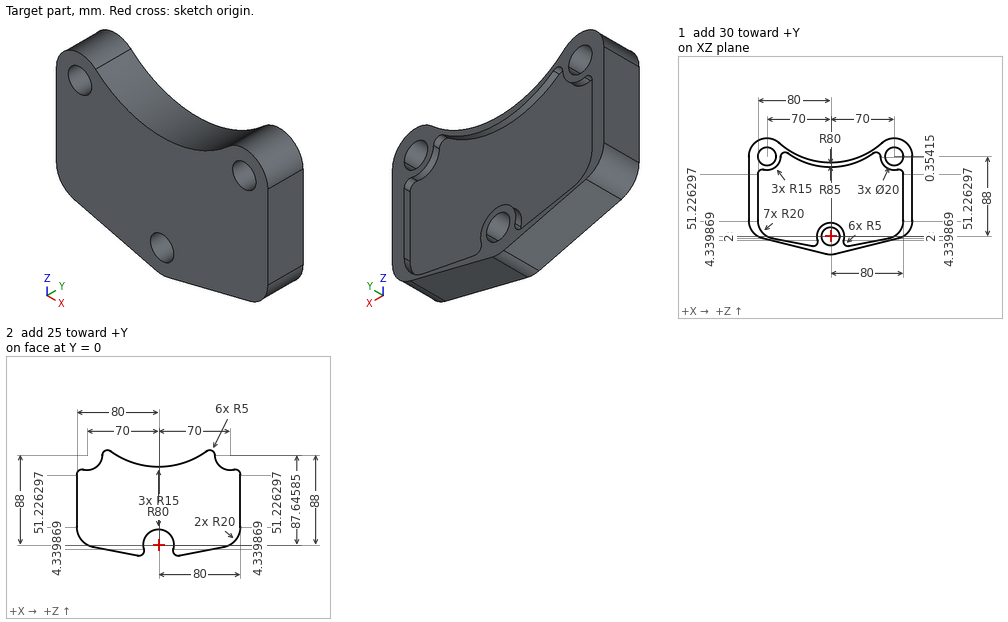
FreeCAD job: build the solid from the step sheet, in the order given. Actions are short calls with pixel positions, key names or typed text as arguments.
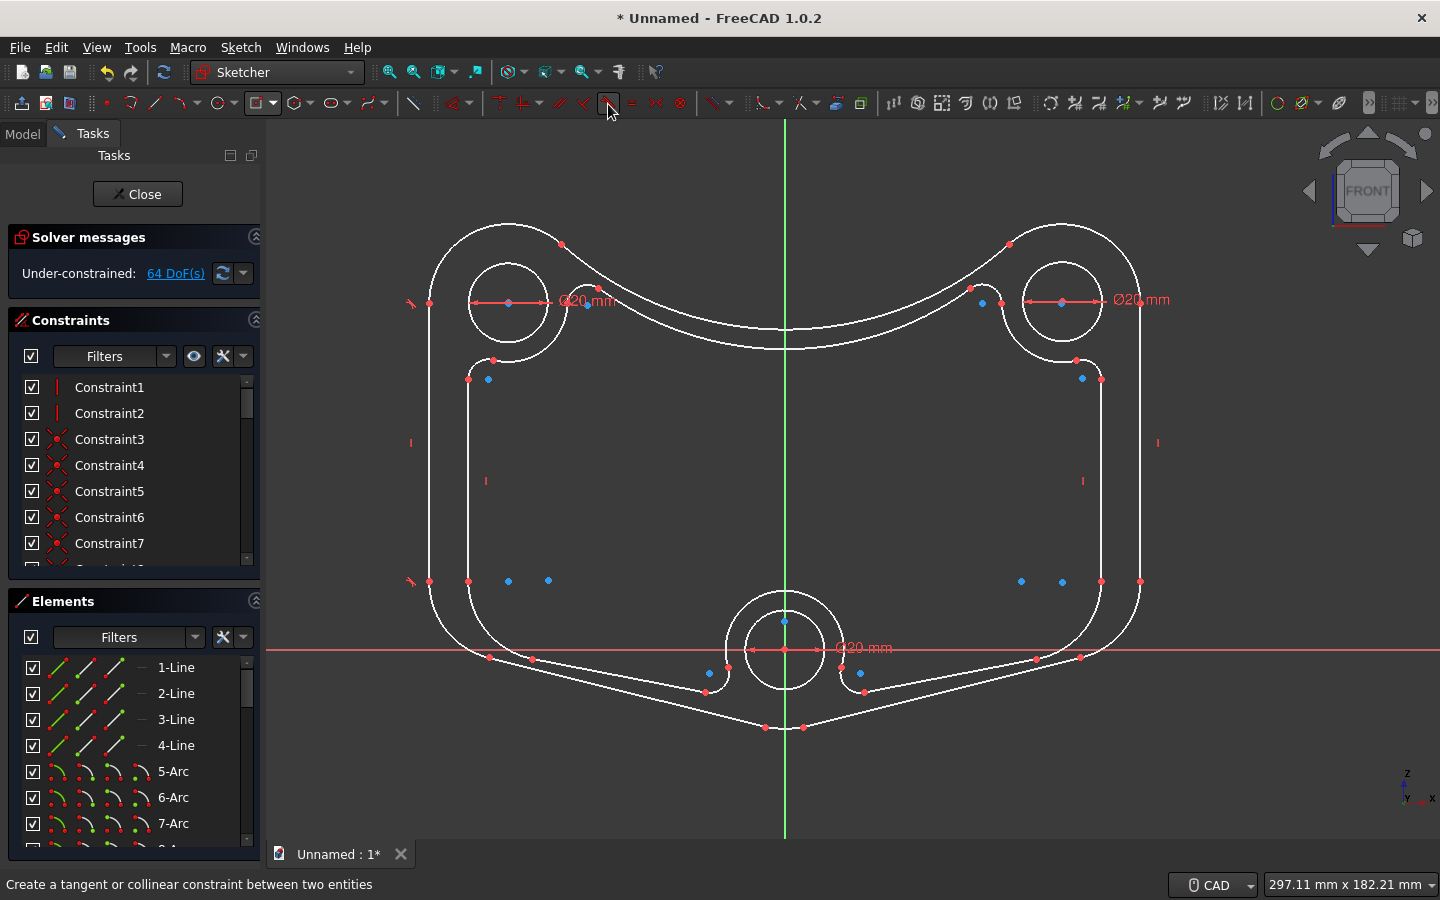
click(1140, 387)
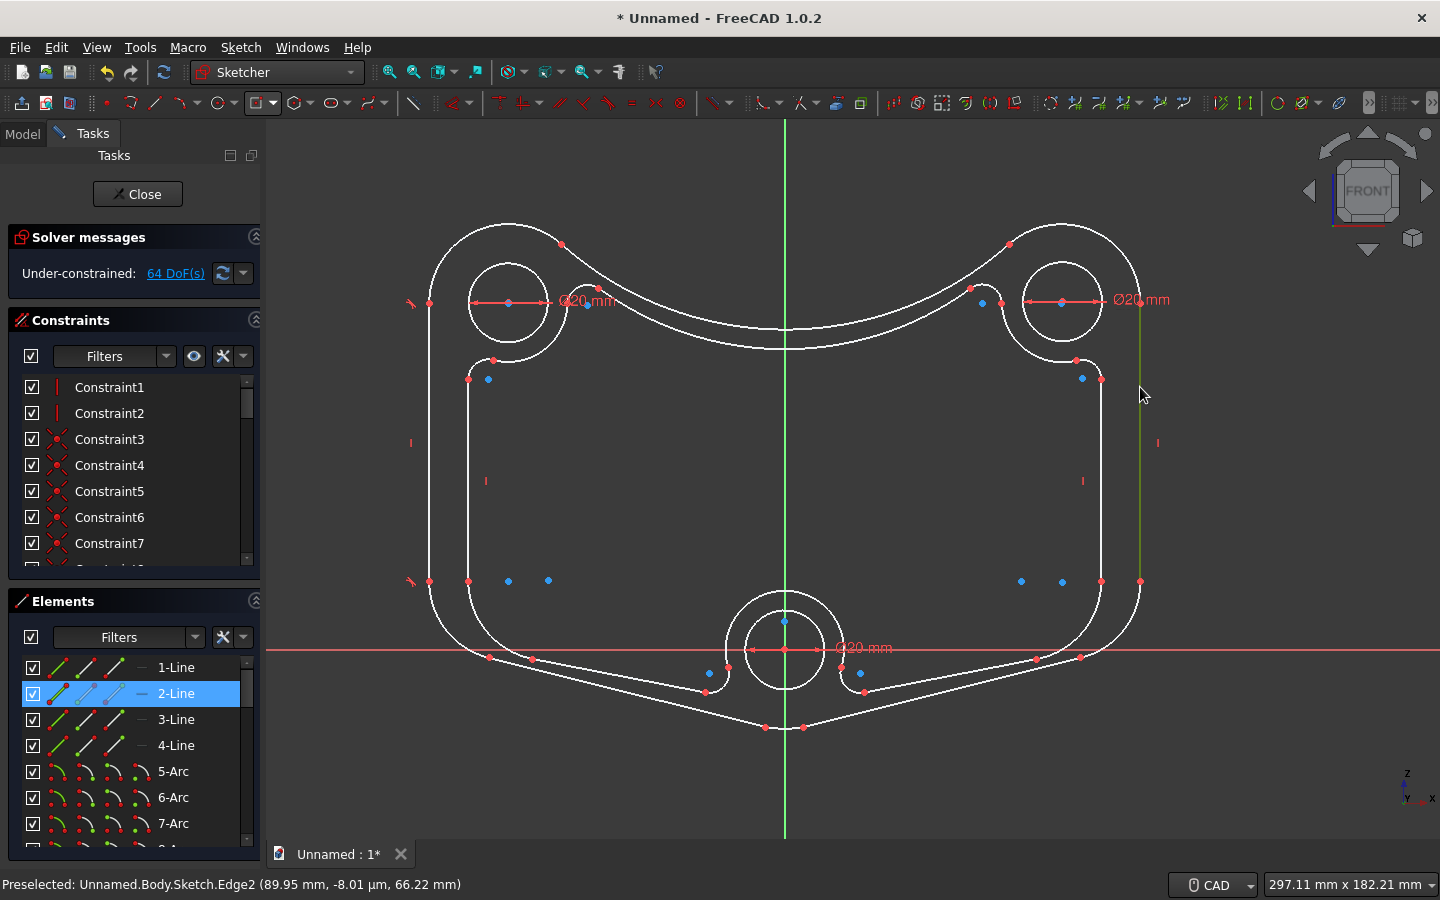
click(1122, 253)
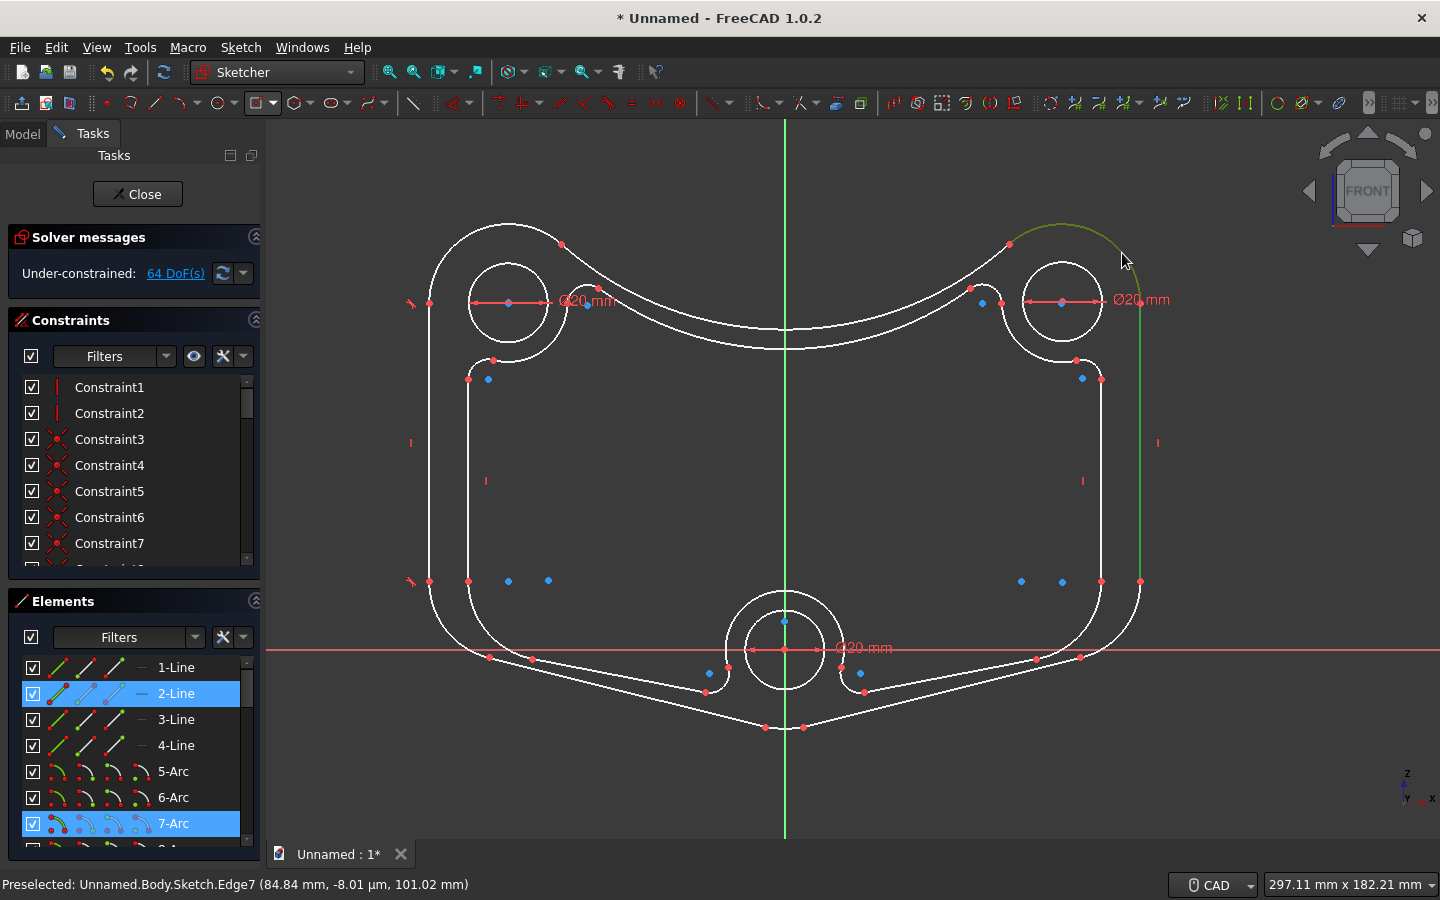
click(608, 104)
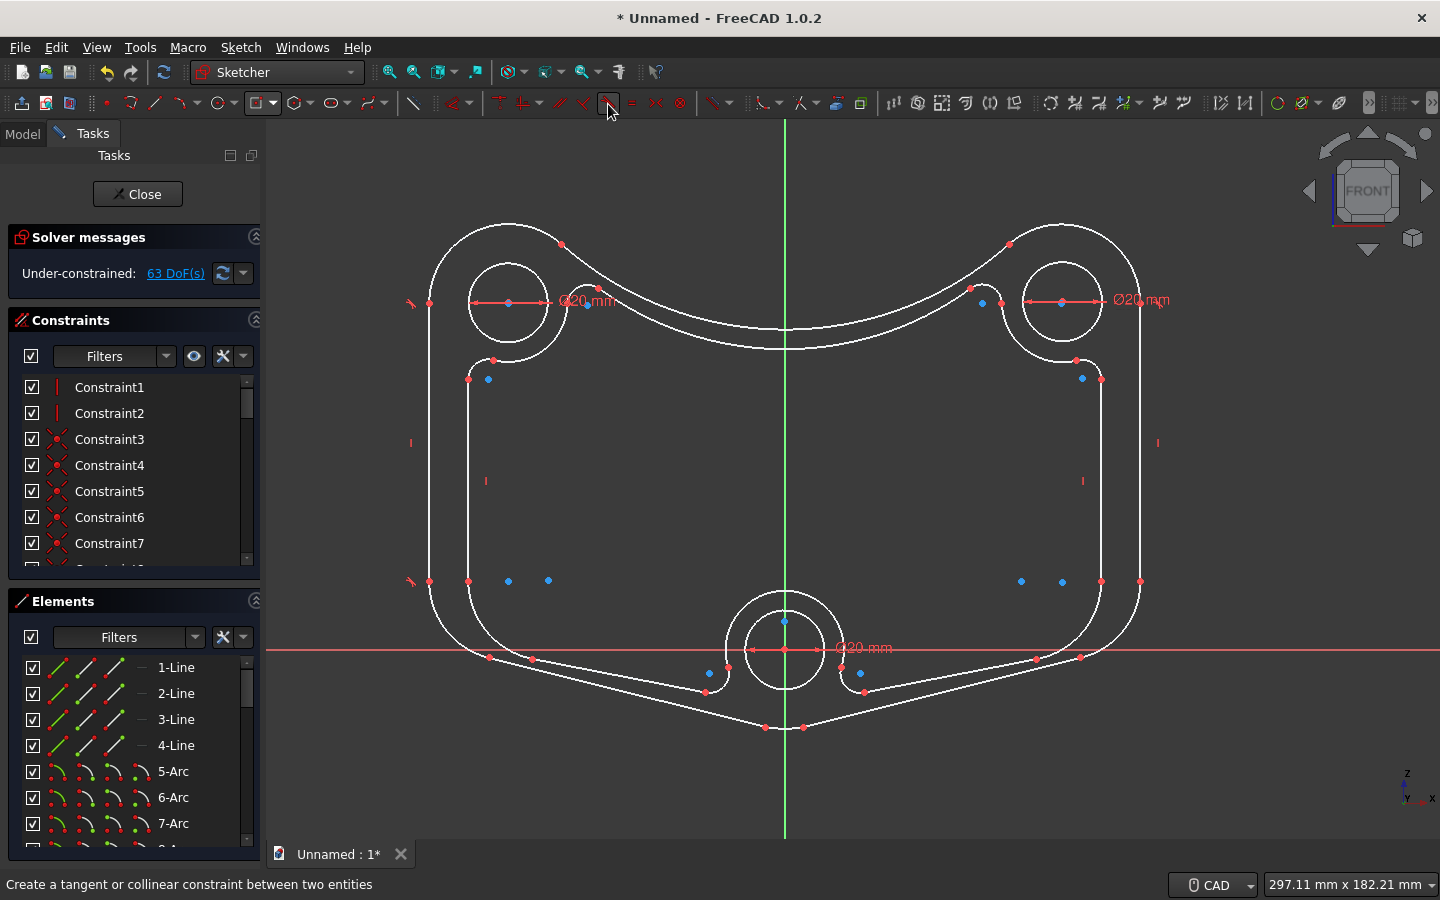
click(1140, 387)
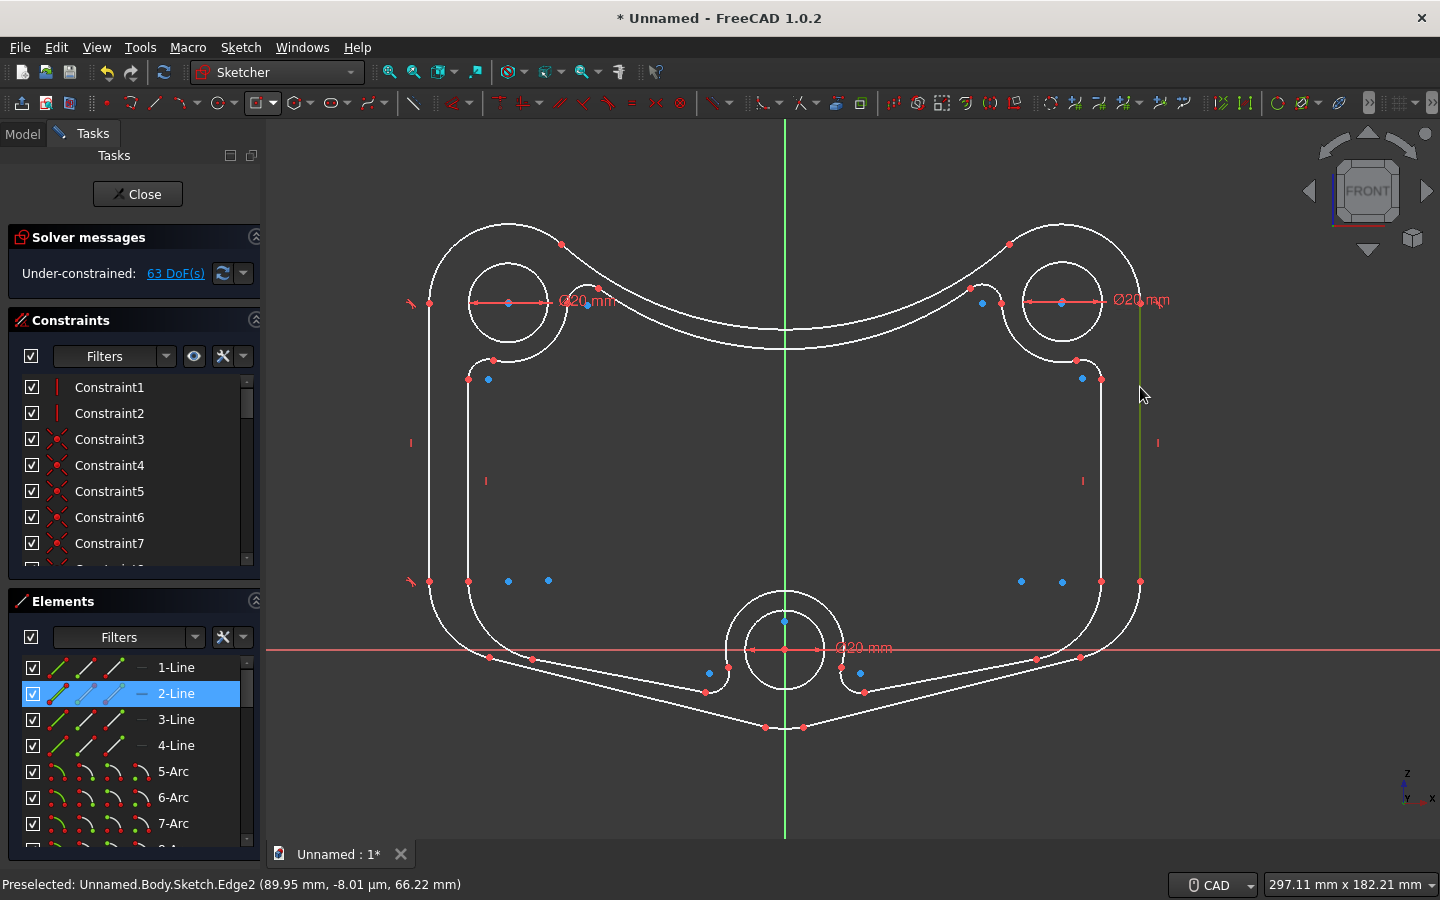
click(1134, 612)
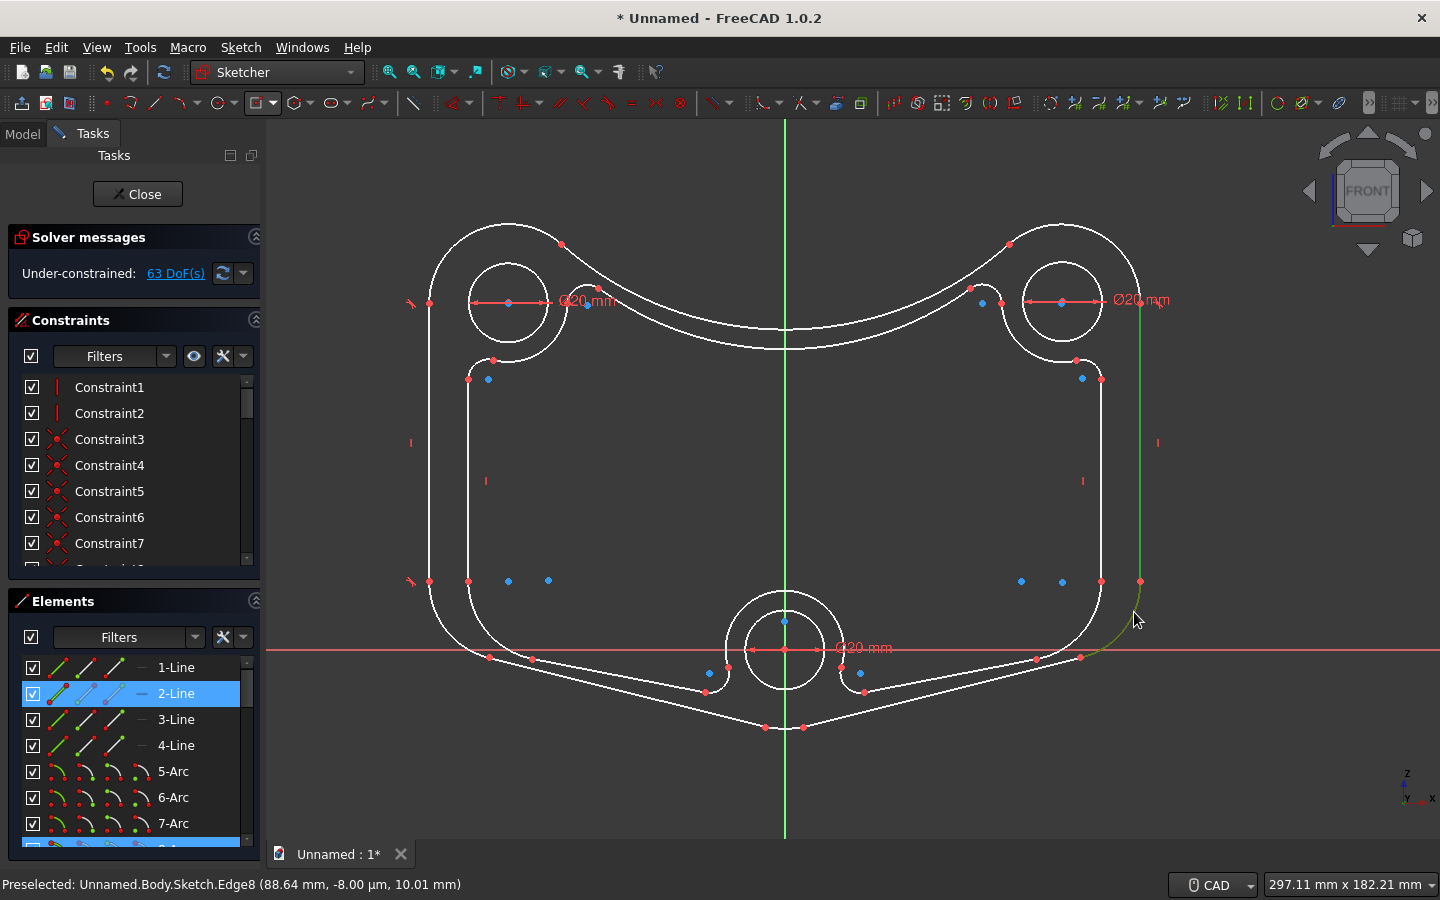
click(608, 104)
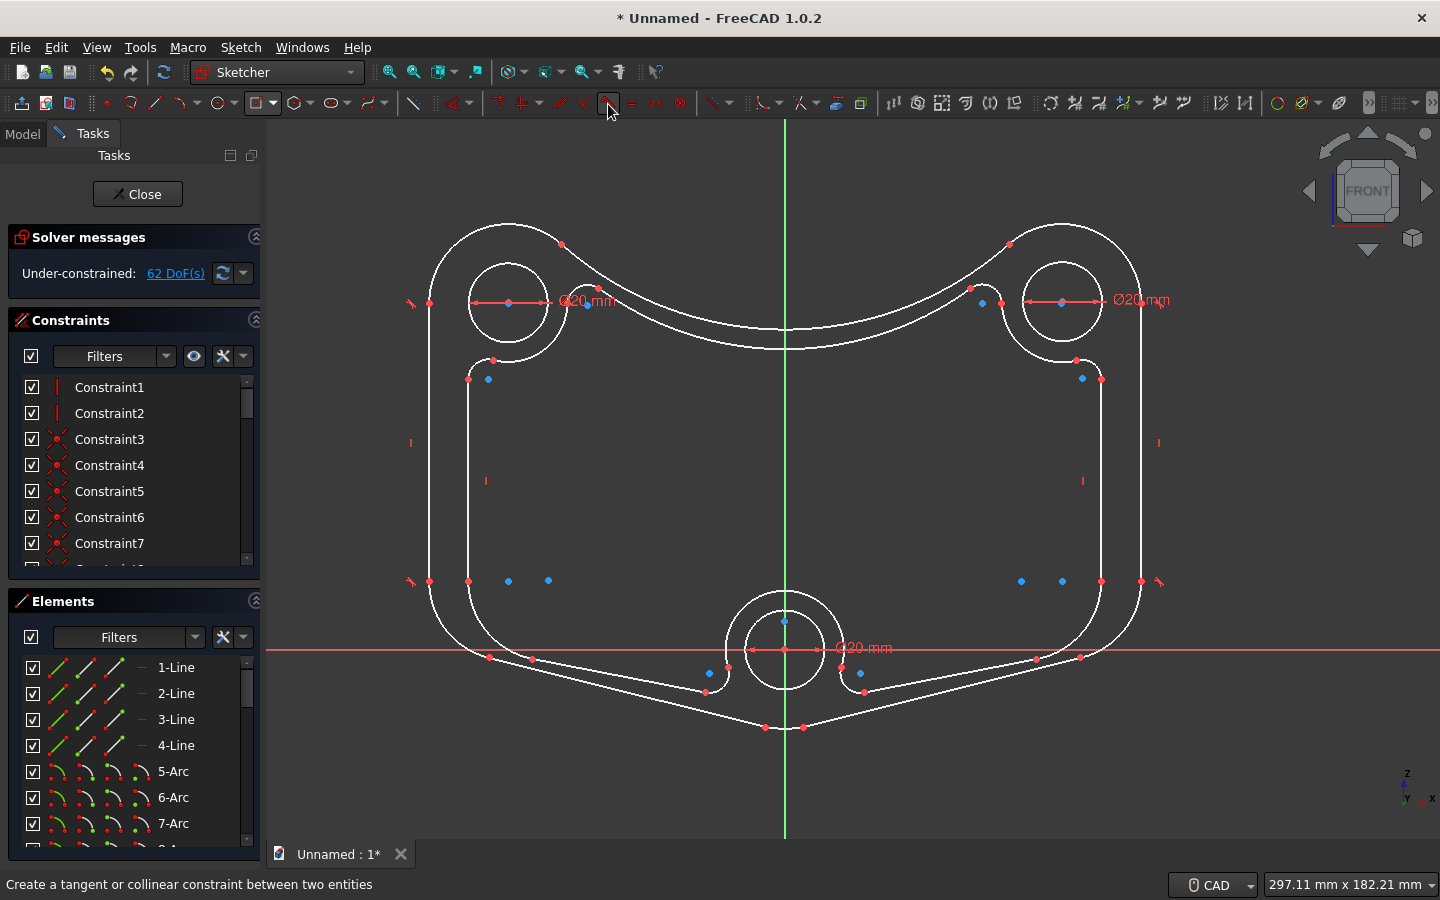
click(998, 679)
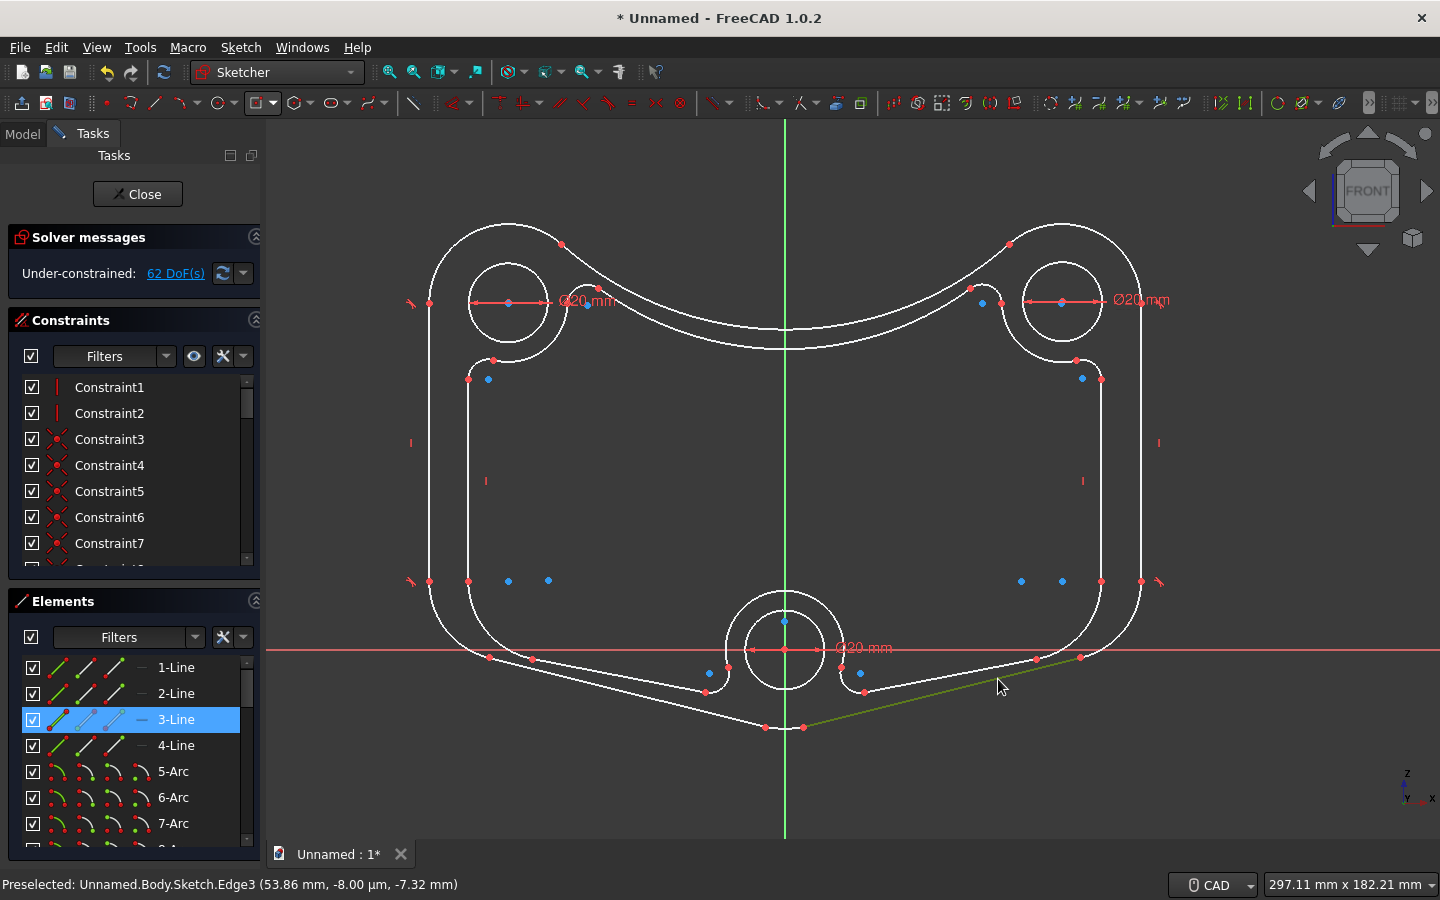
click(1135, 612)